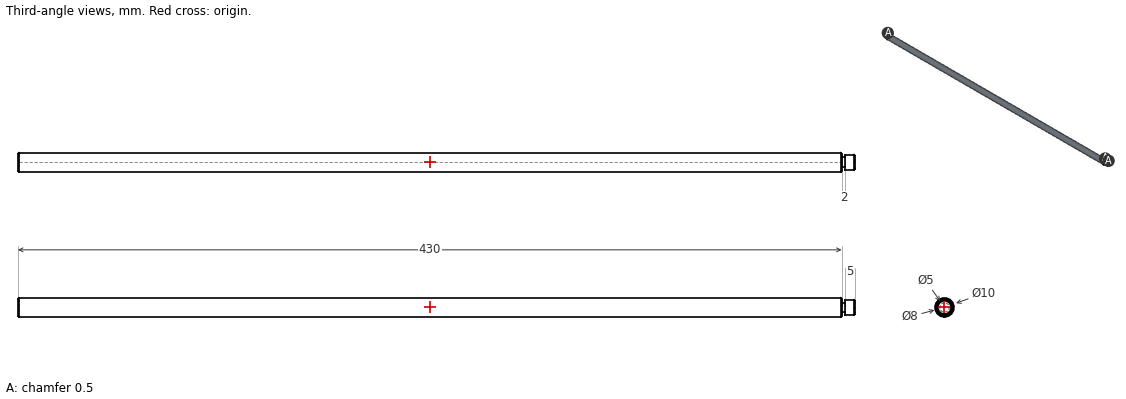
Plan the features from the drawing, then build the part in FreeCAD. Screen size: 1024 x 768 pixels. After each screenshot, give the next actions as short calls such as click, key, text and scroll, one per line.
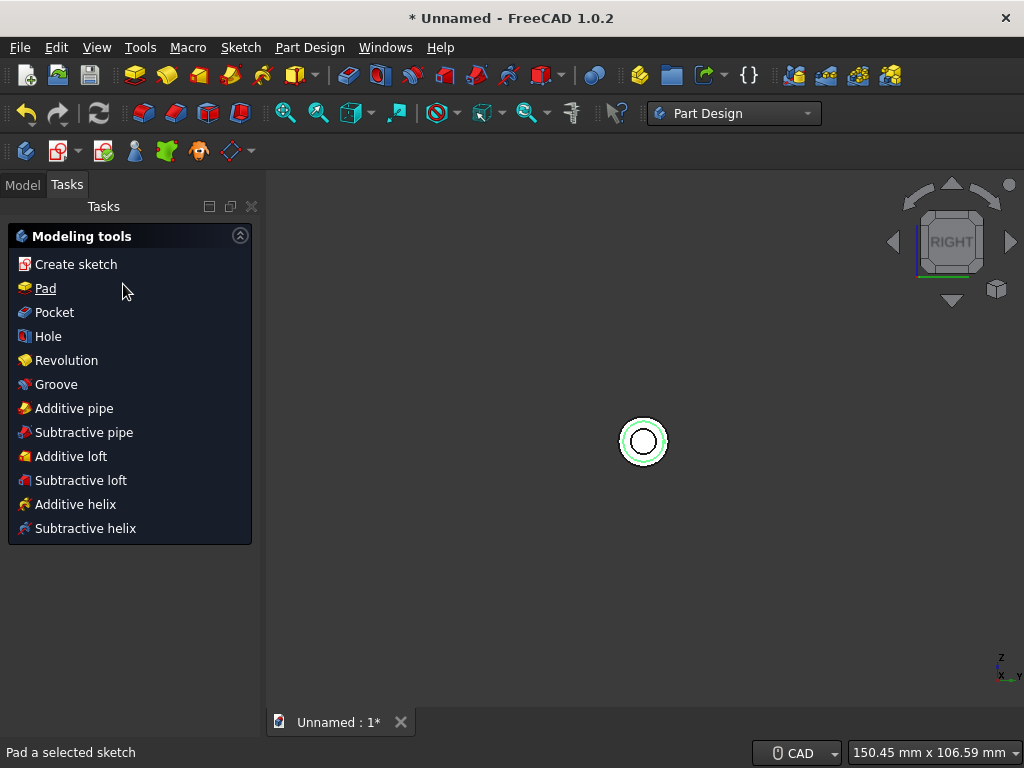
click(136, 76)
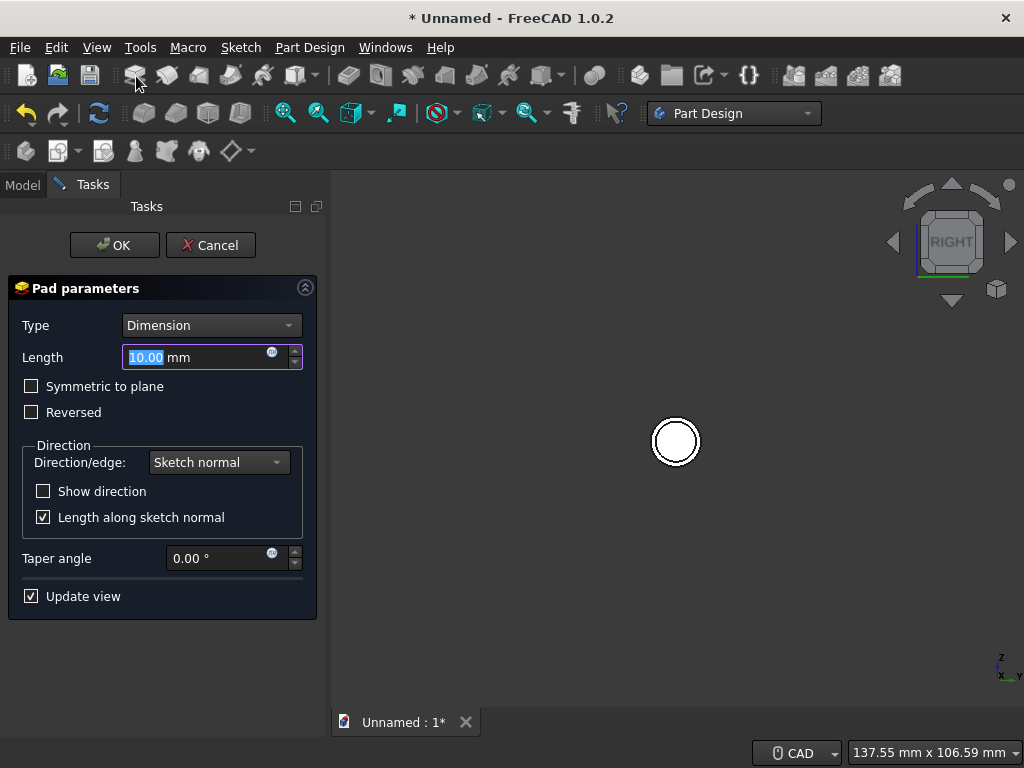
text(5)
key(Tab)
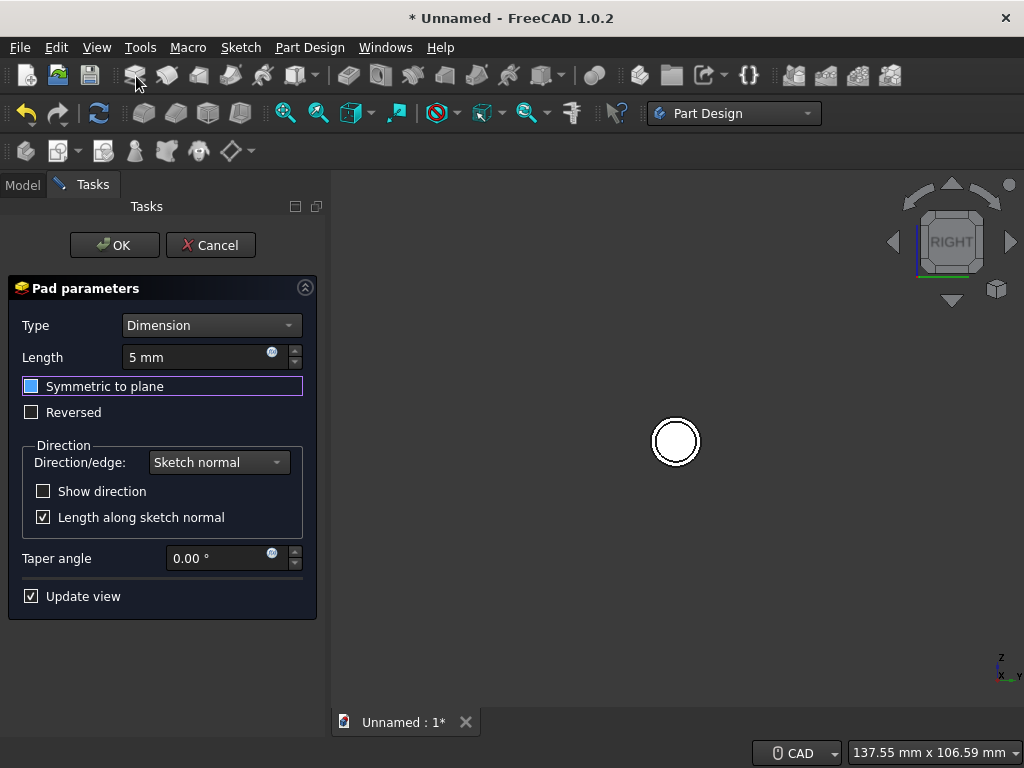
click(115, 245)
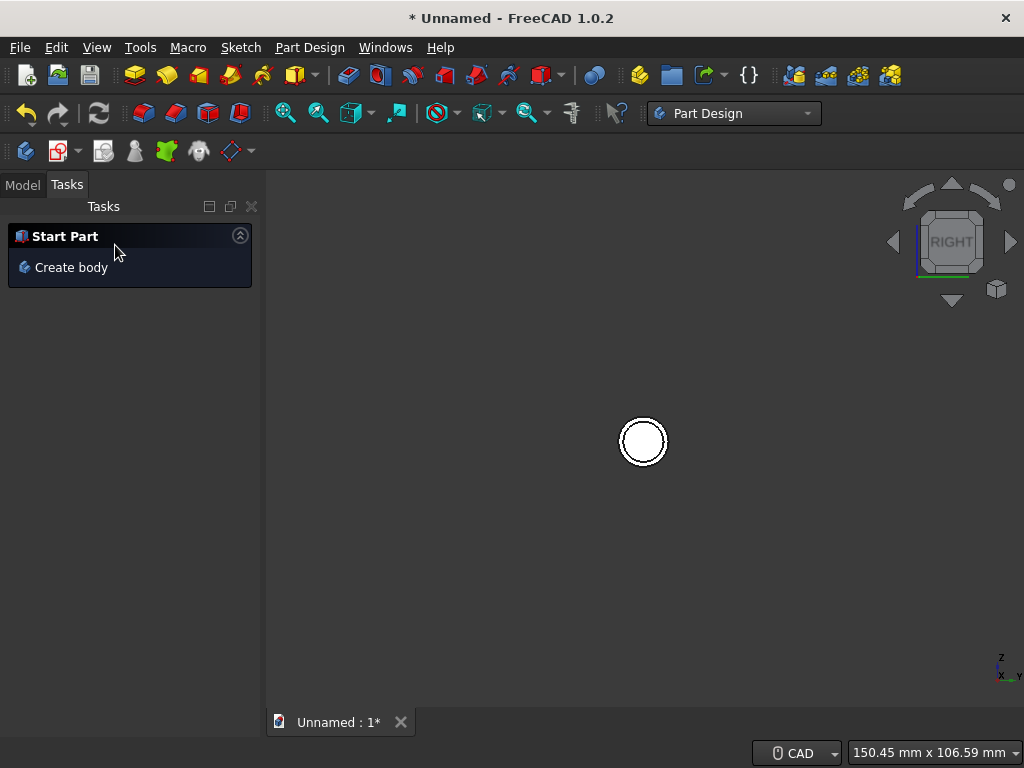
click(286, 114)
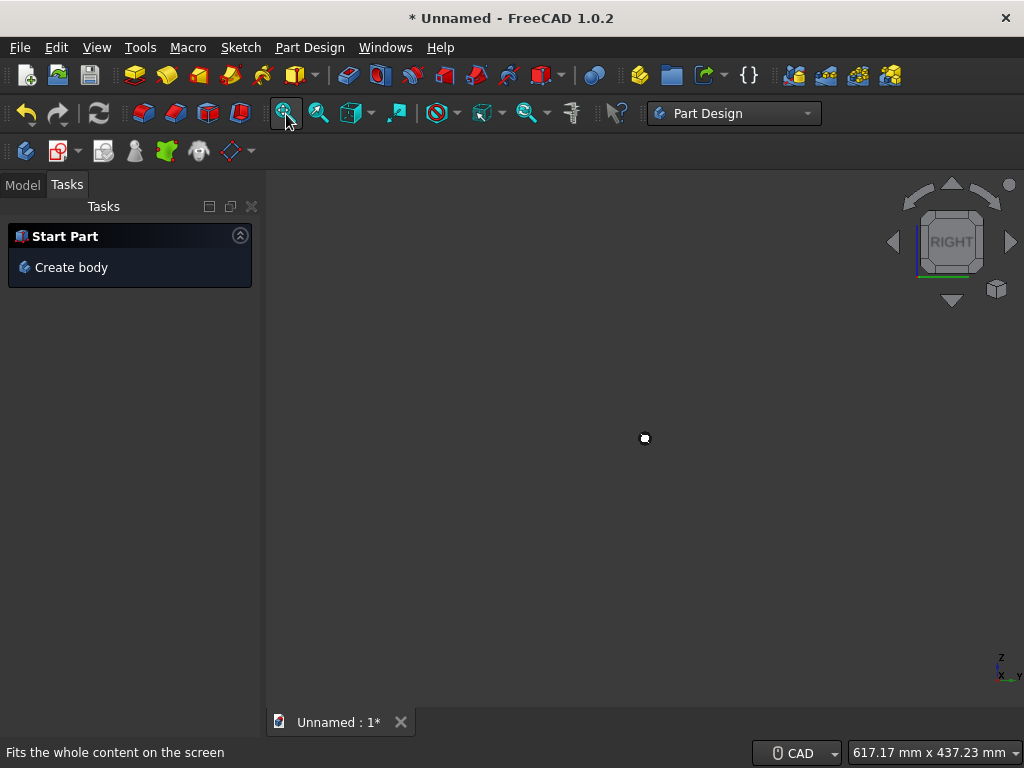
click(640, 437)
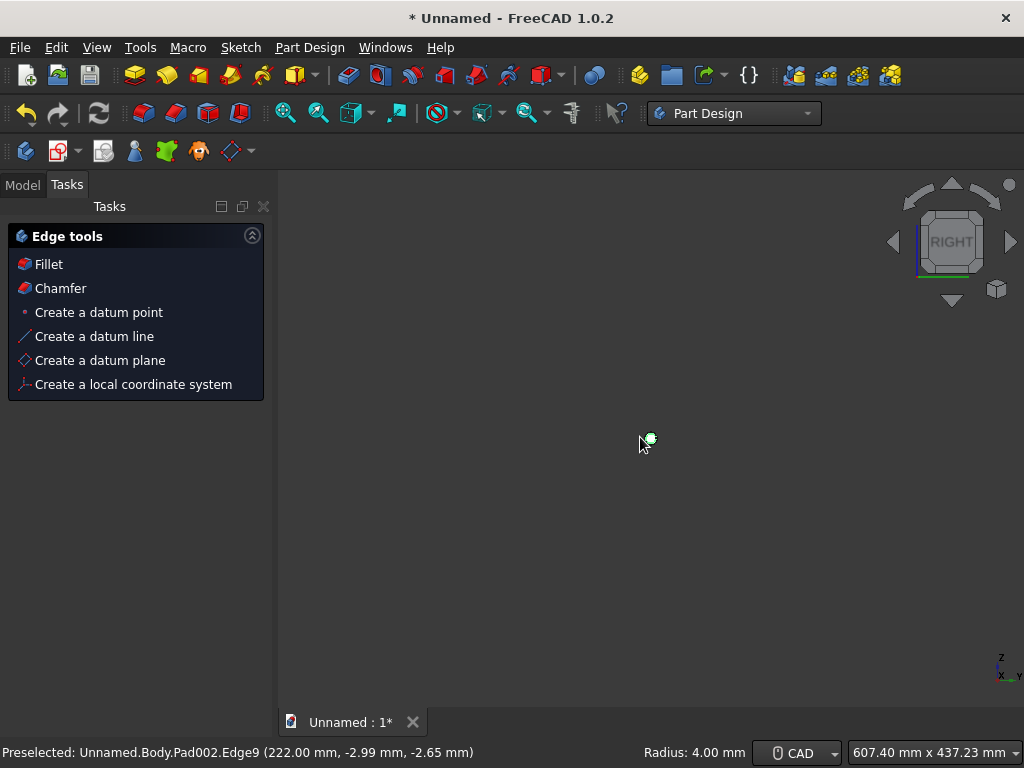
key(0)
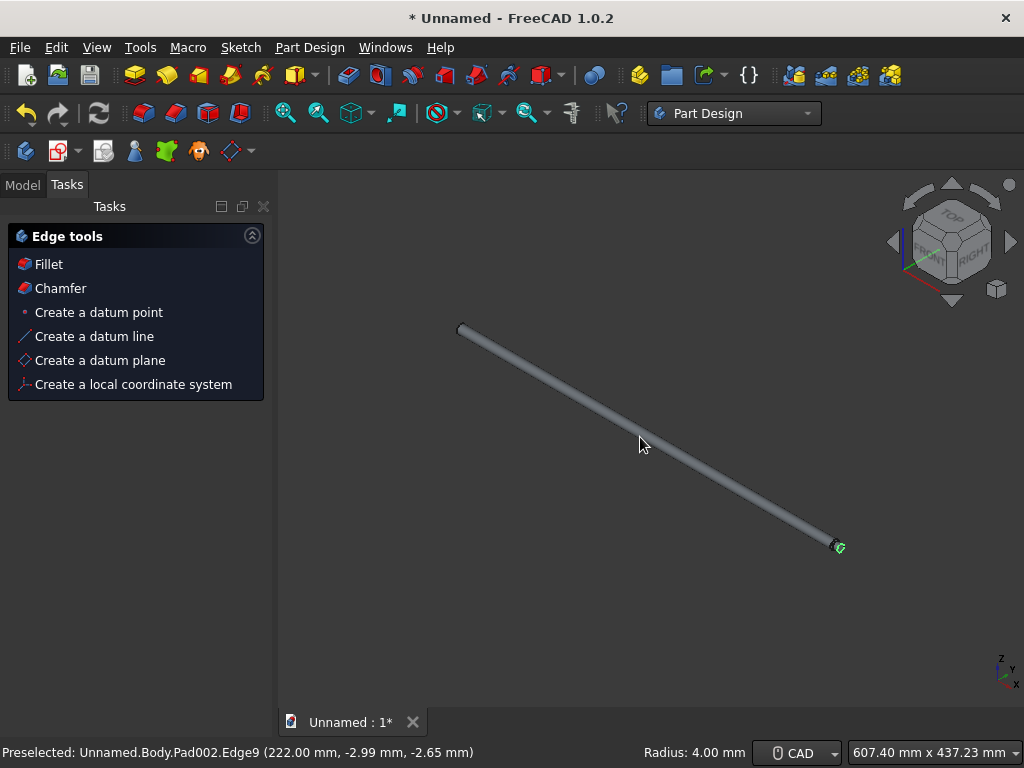
click(463, 322, ctrl)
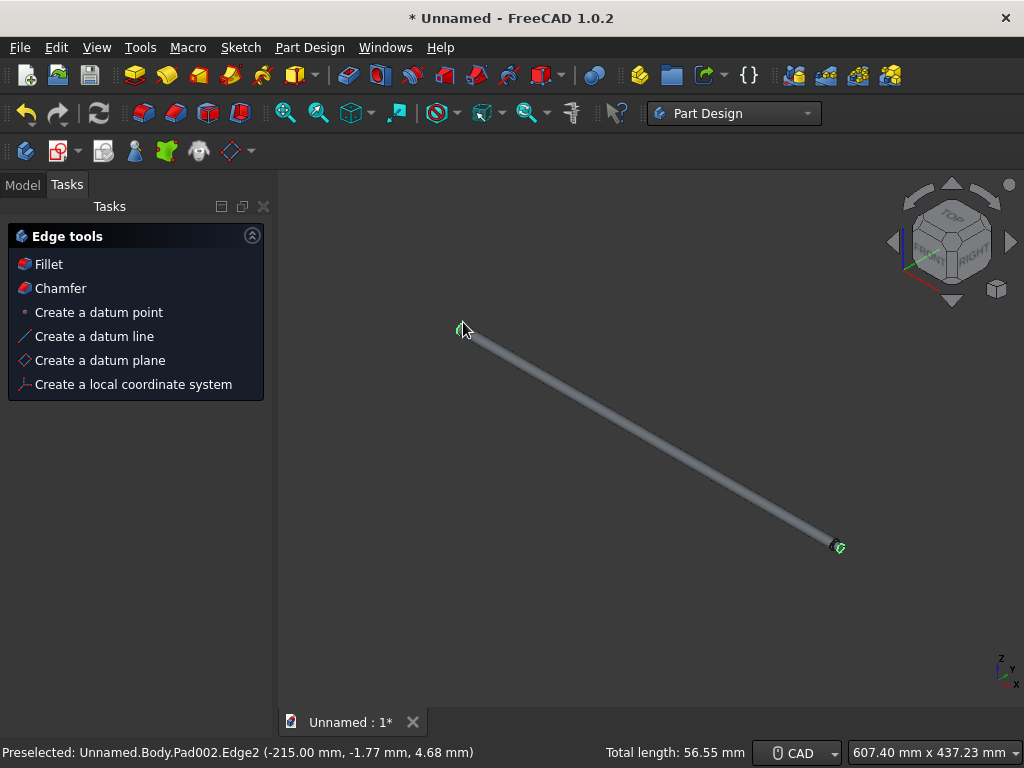
key(2)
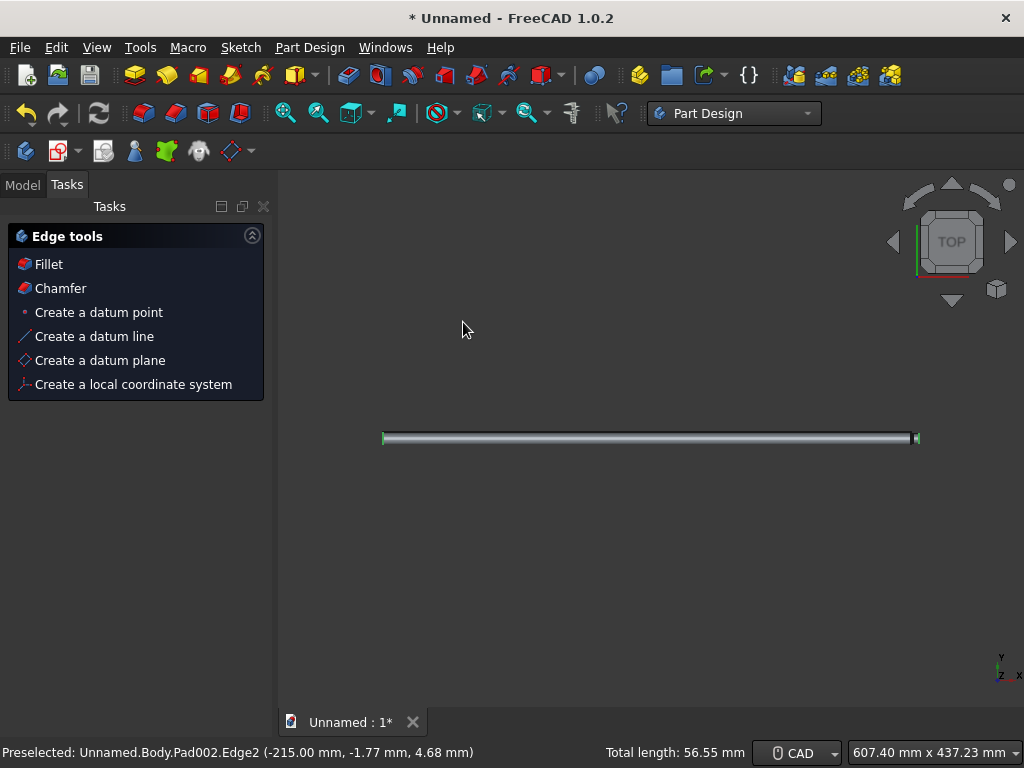
click(911, 444, ctrl)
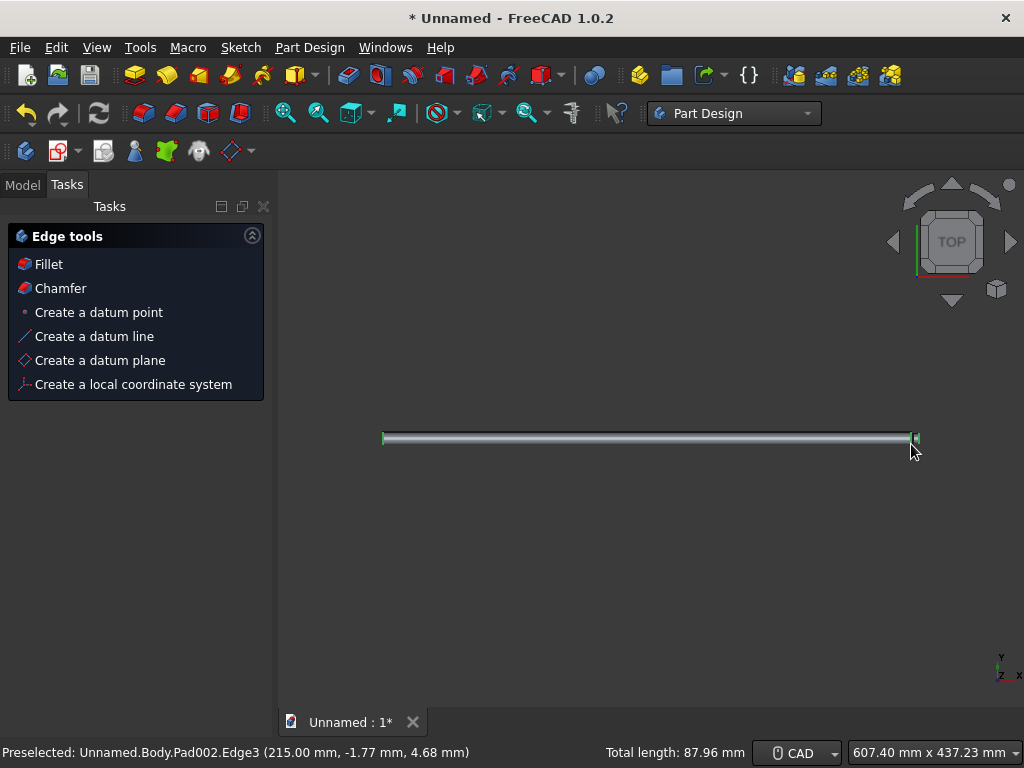
click(176, 114)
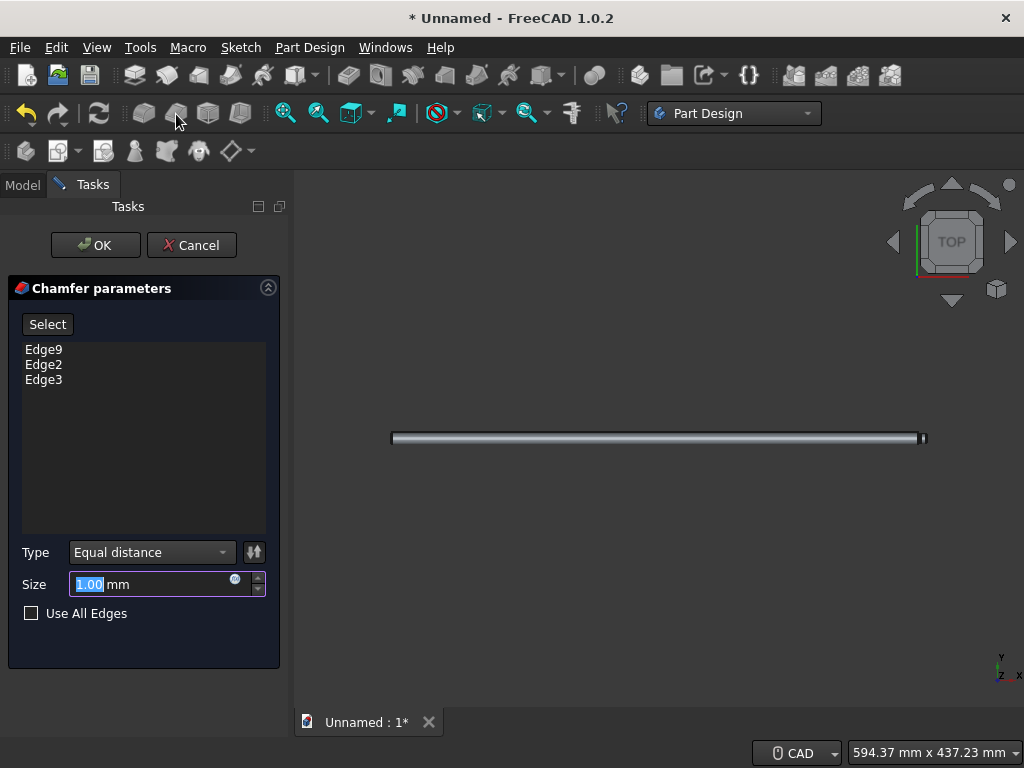
text(0.5)
key(Tab)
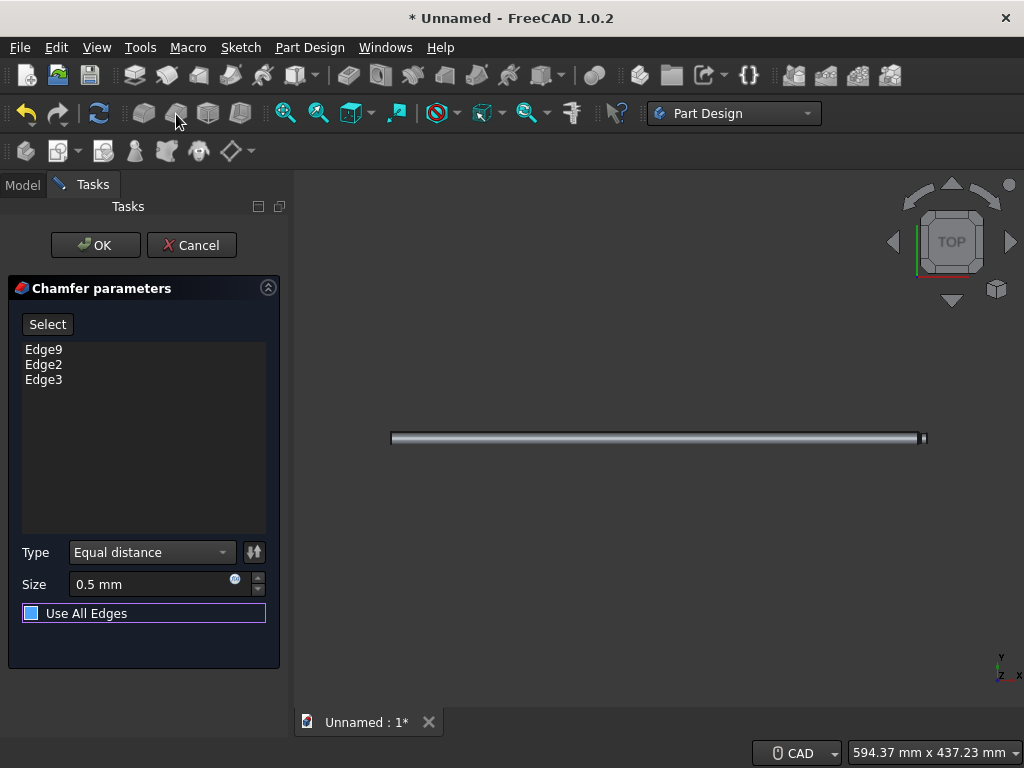
click(96, 245)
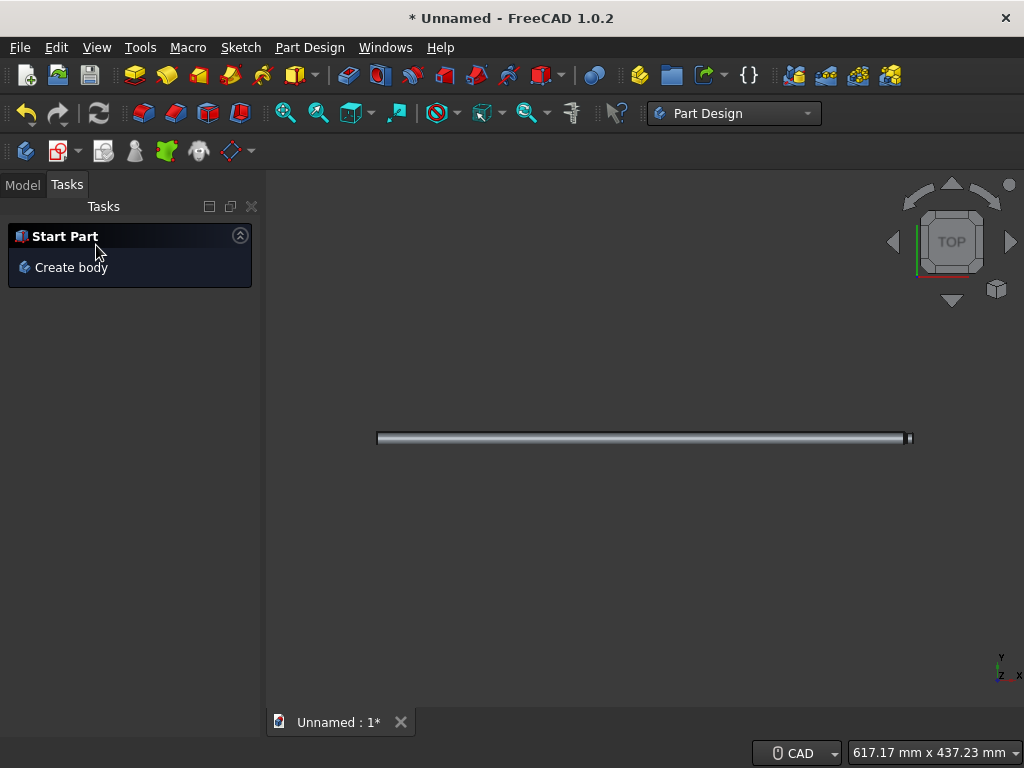
key(0)